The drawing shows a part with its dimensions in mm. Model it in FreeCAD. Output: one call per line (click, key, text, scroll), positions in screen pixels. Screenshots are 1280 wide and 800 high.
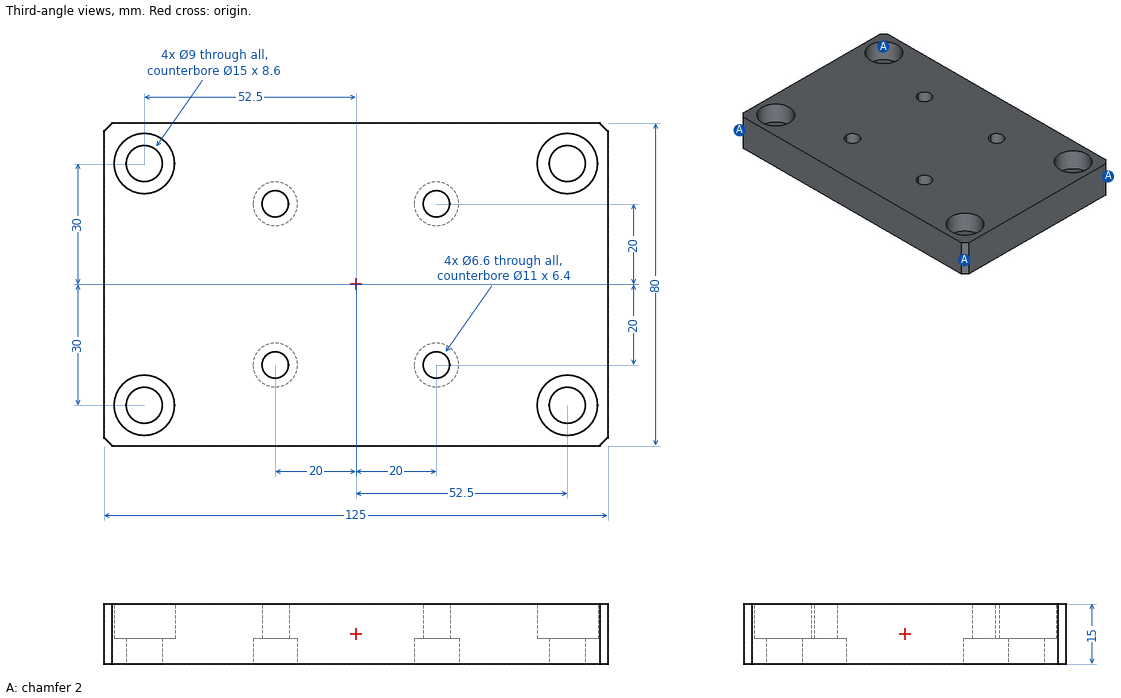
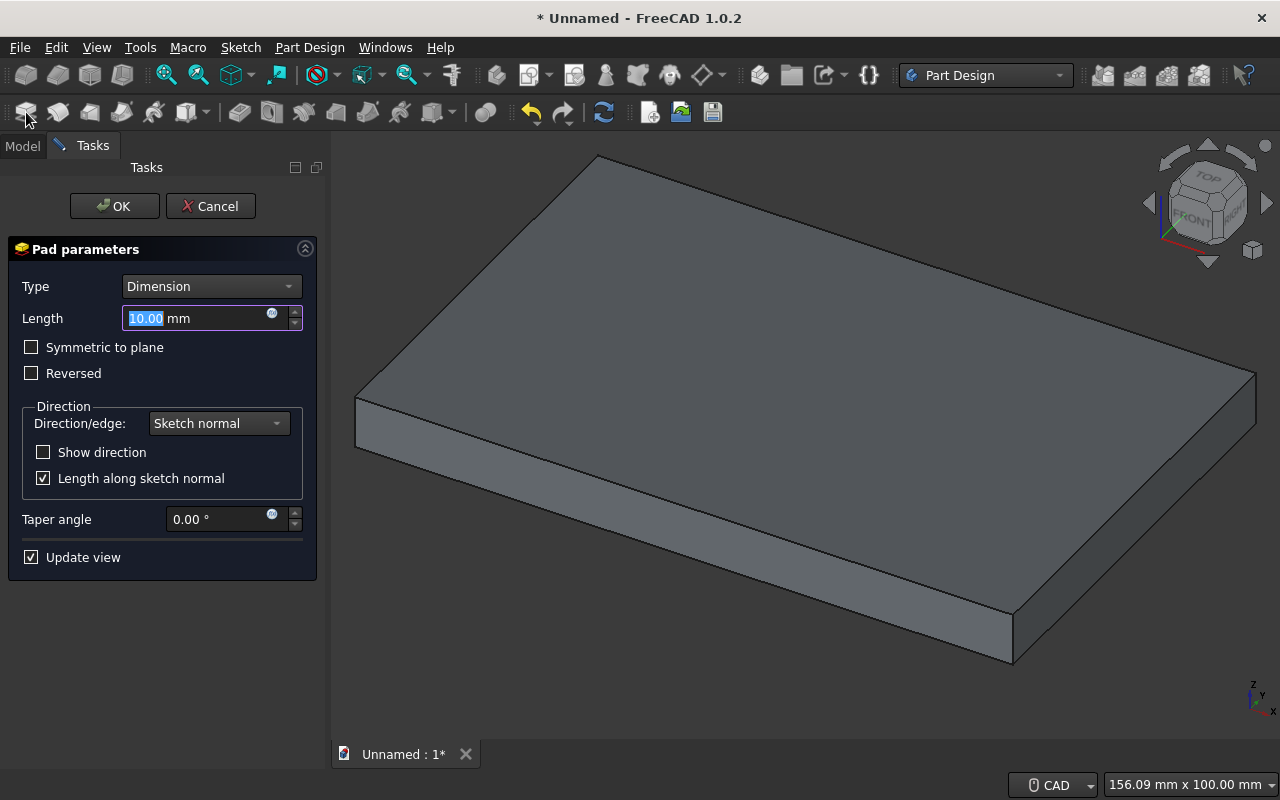
text(15)
key(Tab)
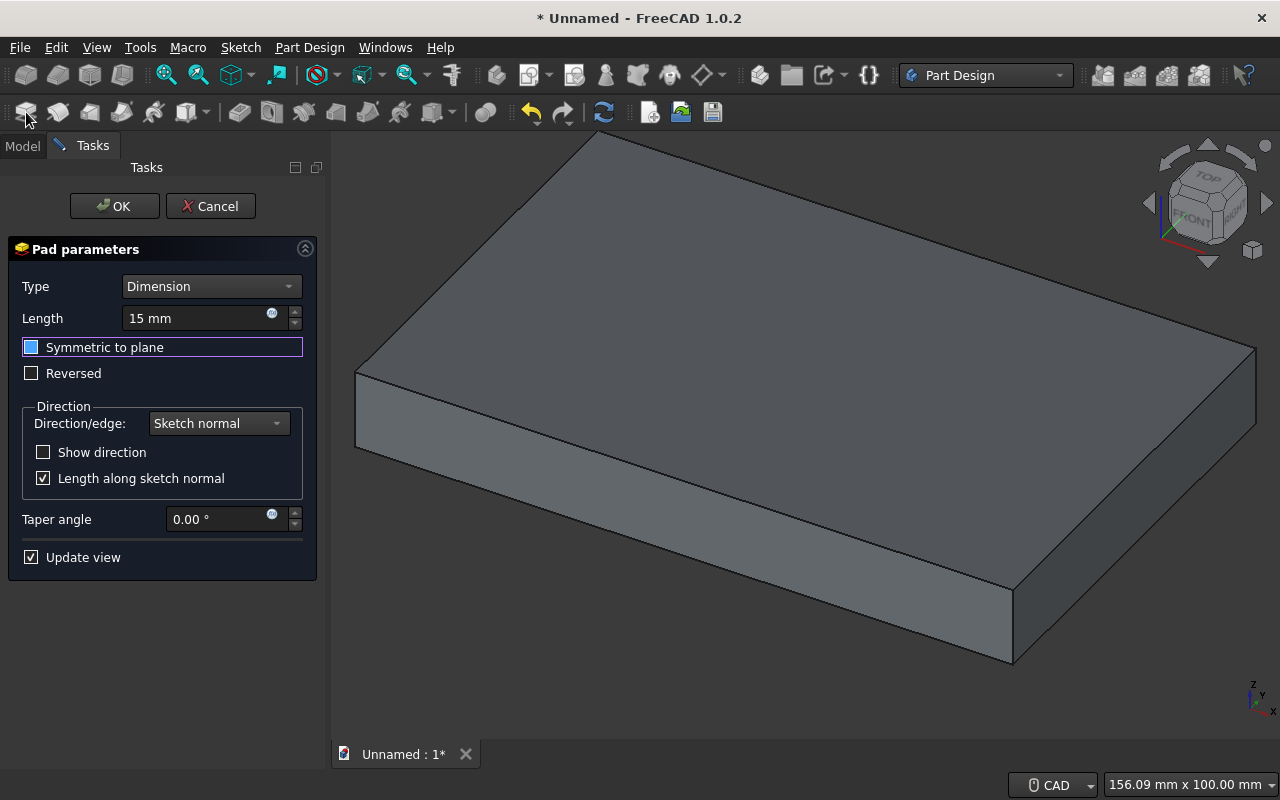
click(30, 347)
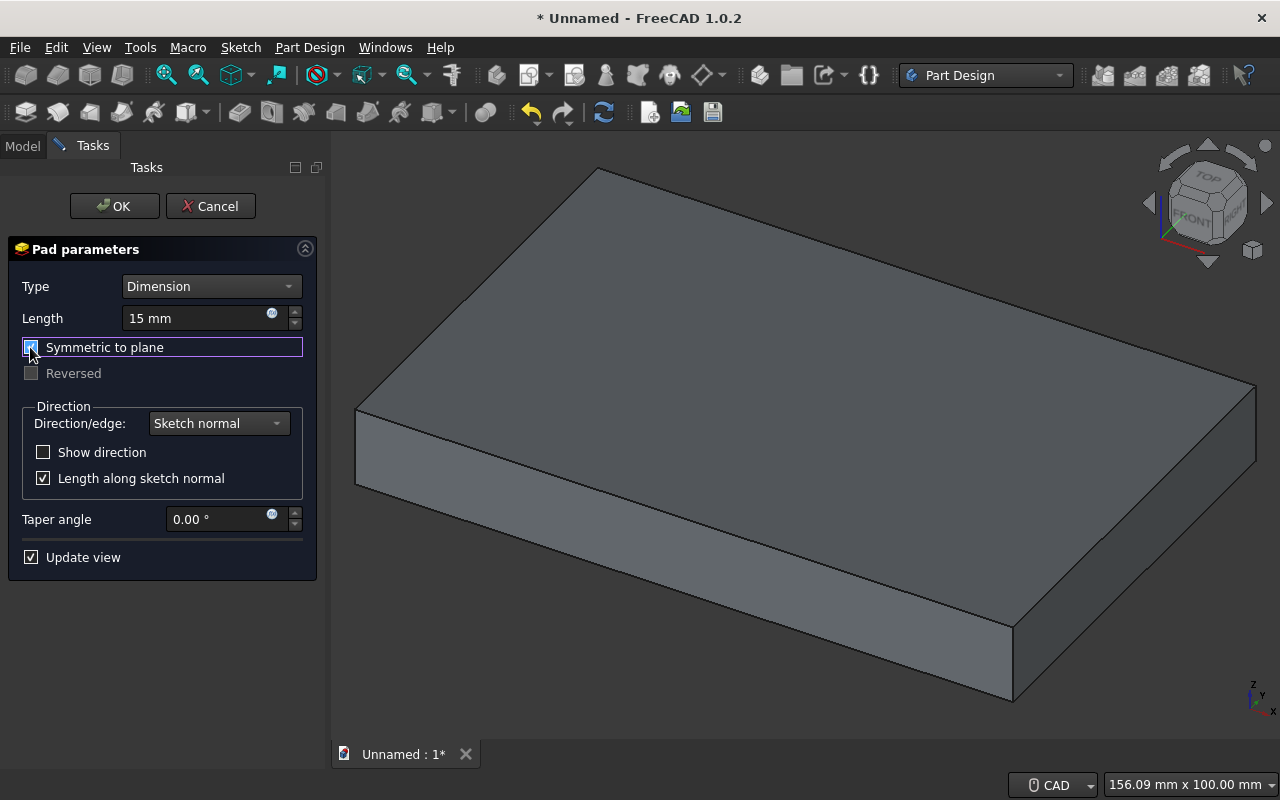
click(115, 206)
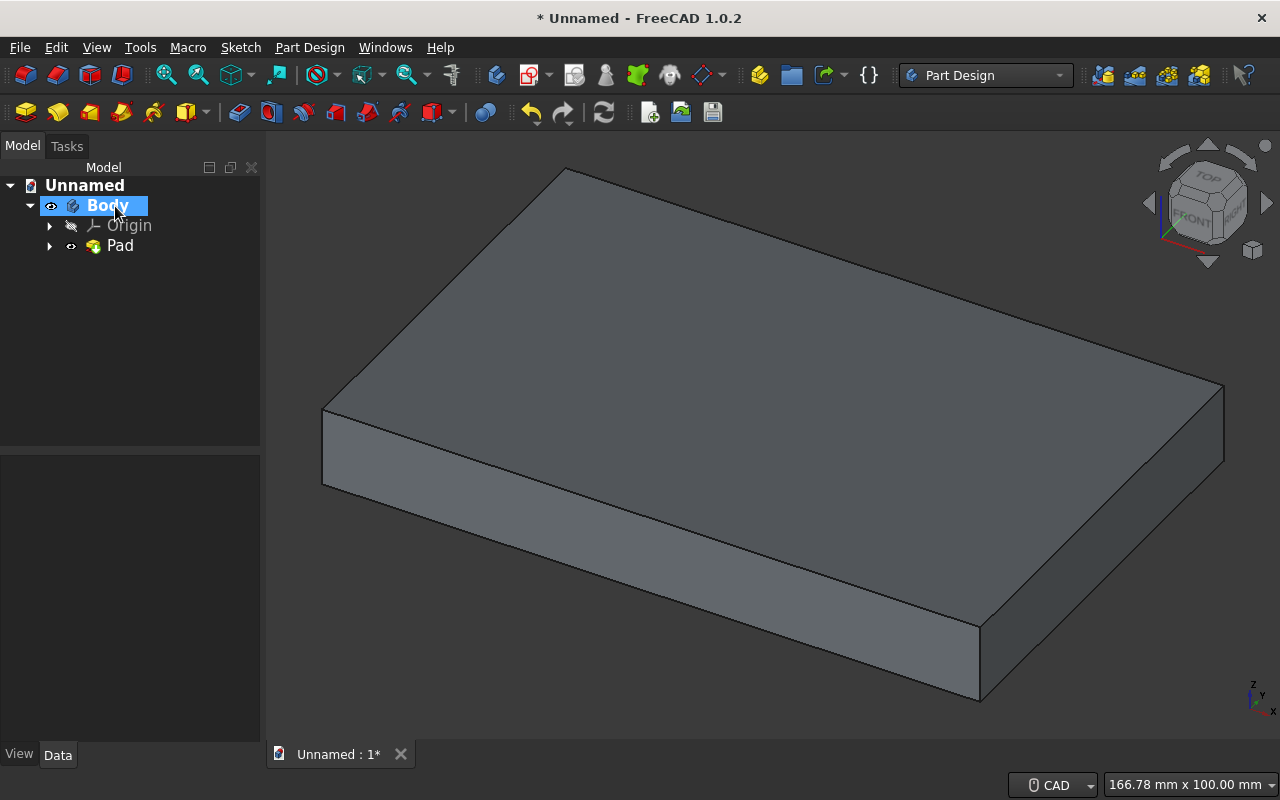
click(867, 428)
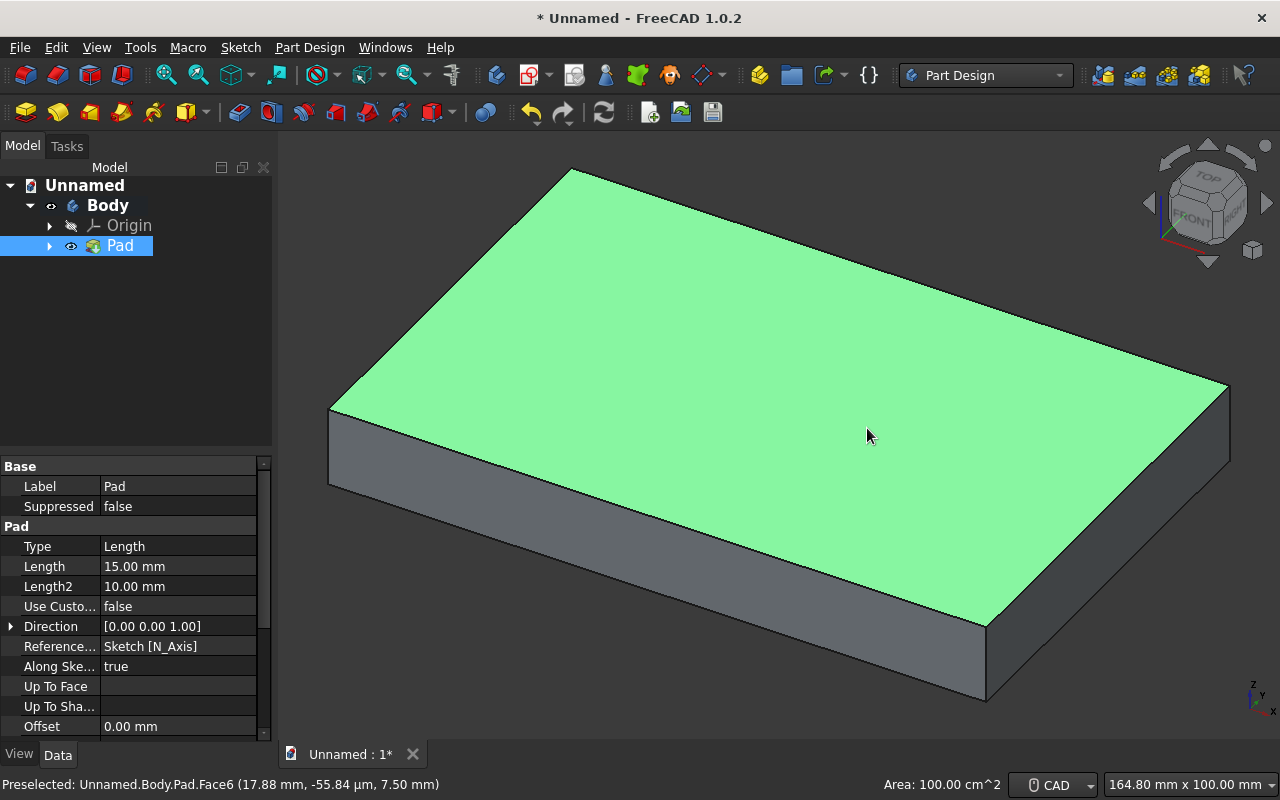
click(530, 76)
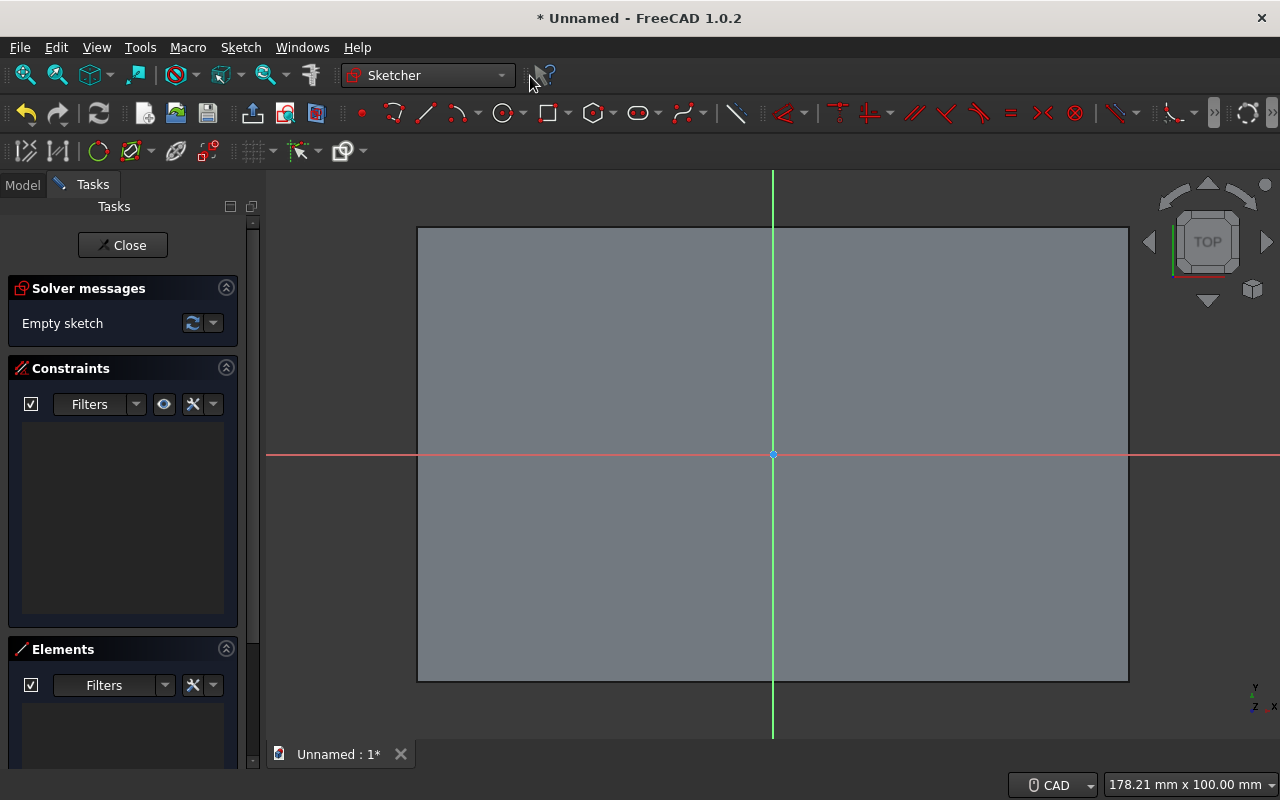
scroll(395, 455, down, 1)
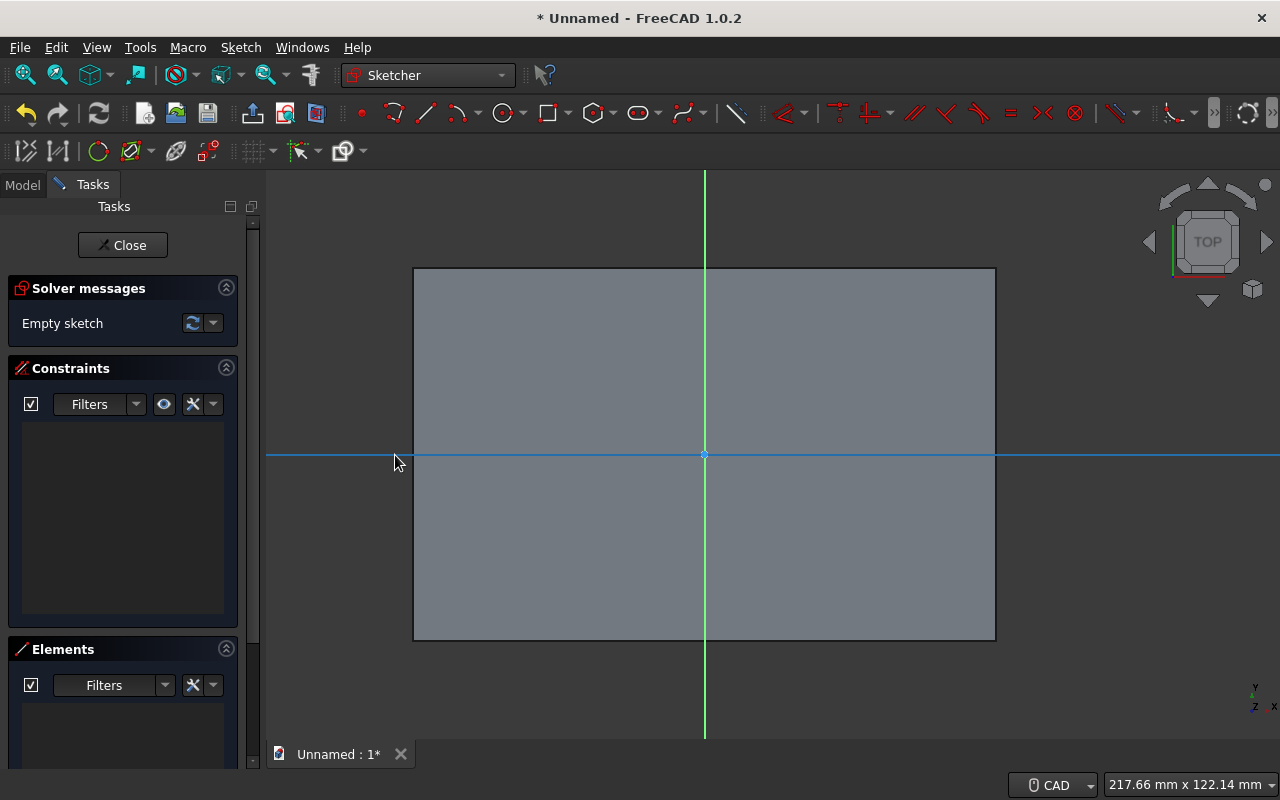
key(g)
key(c)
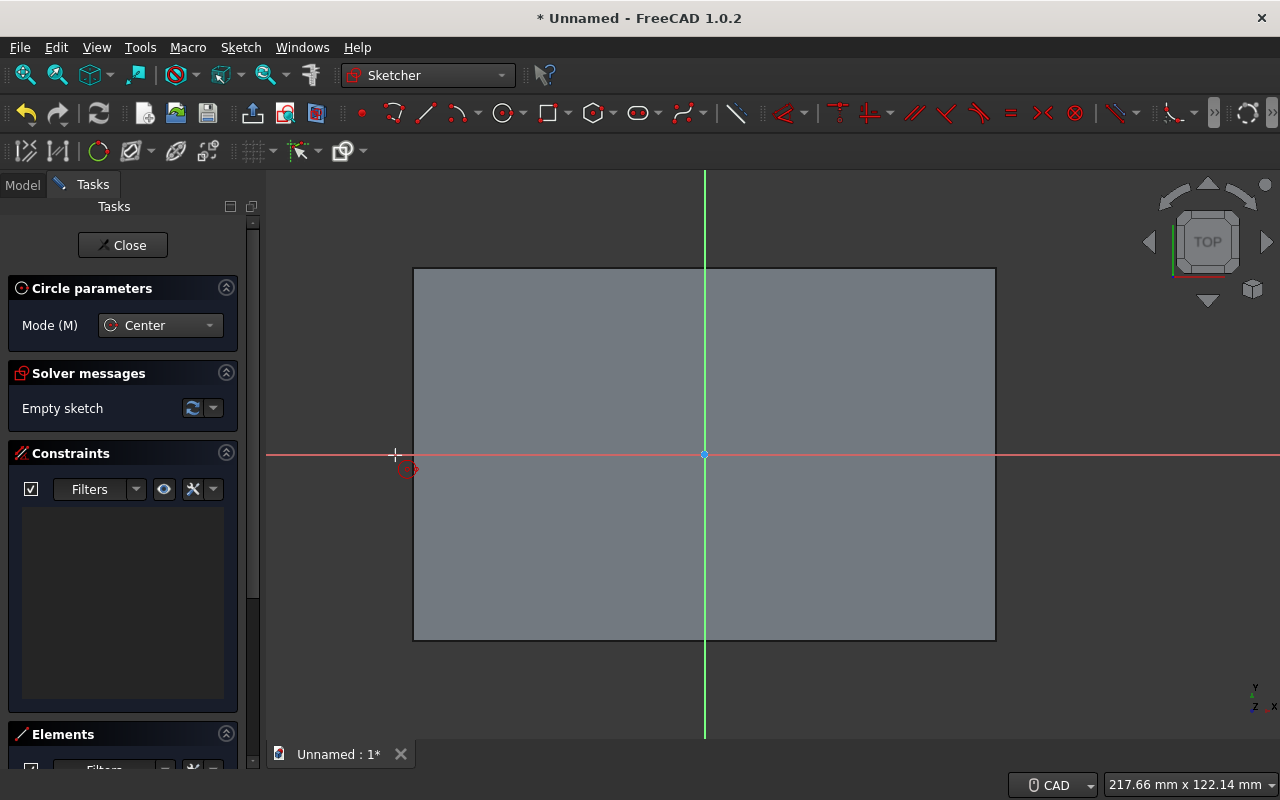
click(460, 315)
move(475, 300)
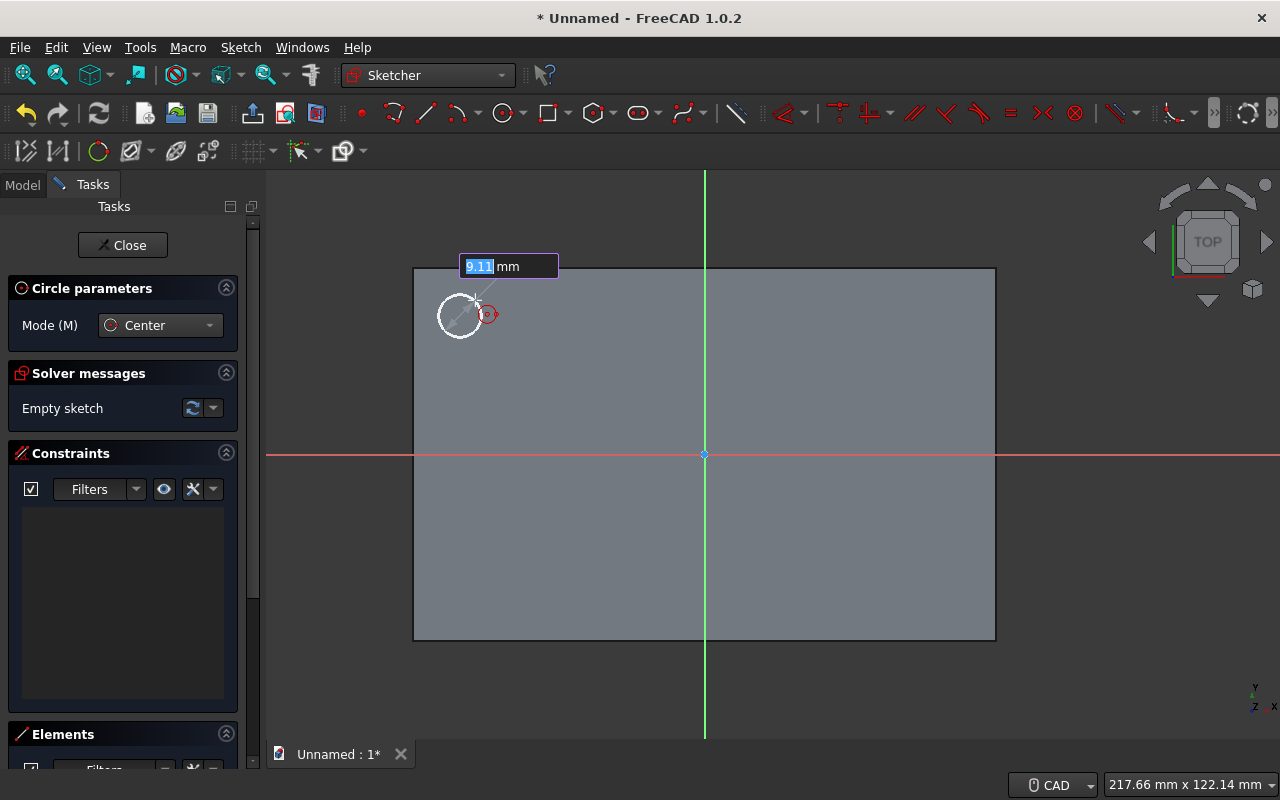
text(9)
key(Return)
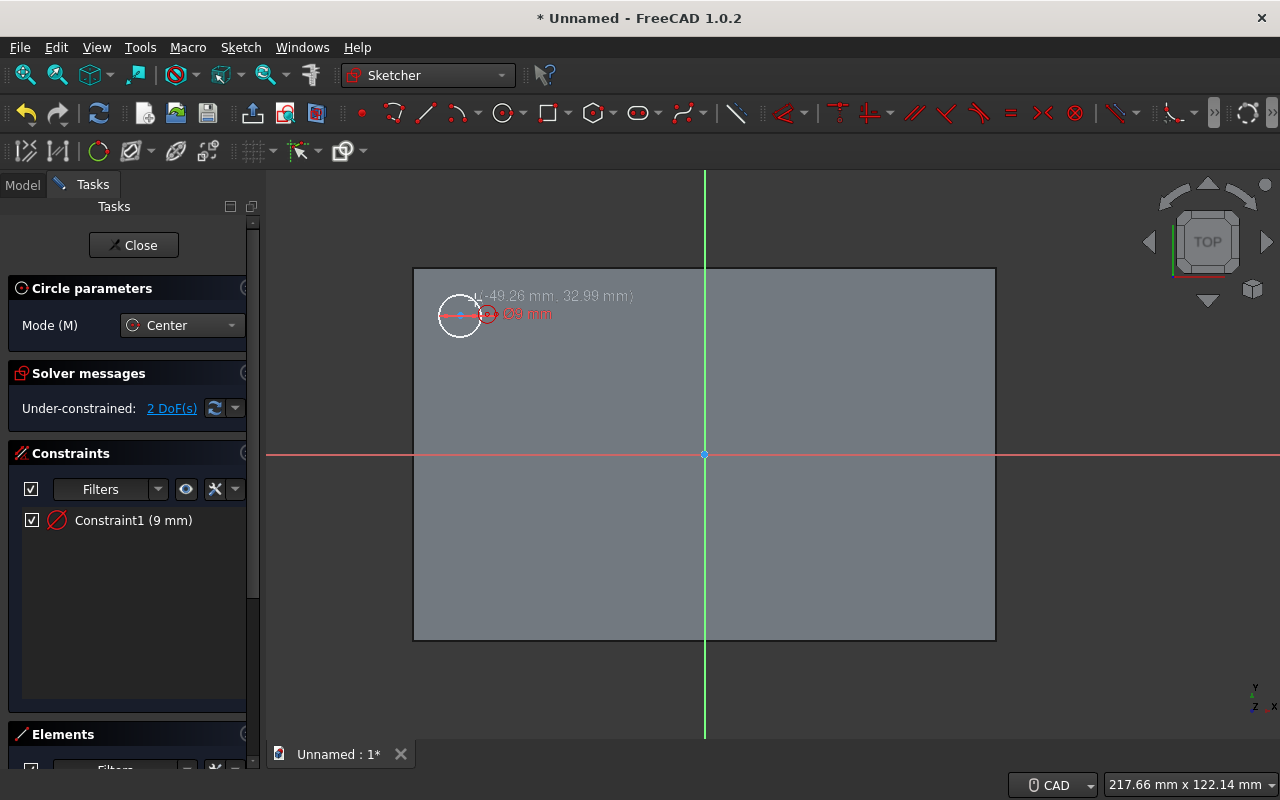
click(460, 594)
move(475, 580)